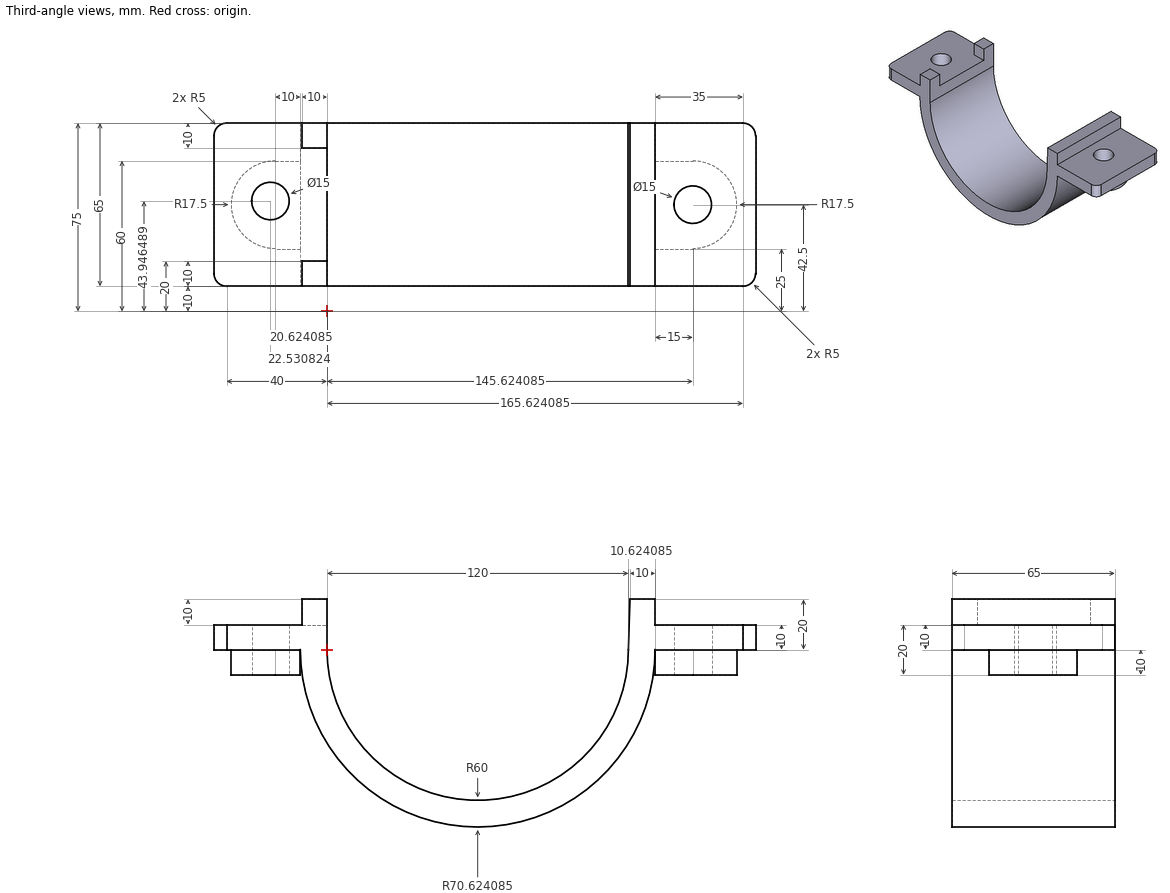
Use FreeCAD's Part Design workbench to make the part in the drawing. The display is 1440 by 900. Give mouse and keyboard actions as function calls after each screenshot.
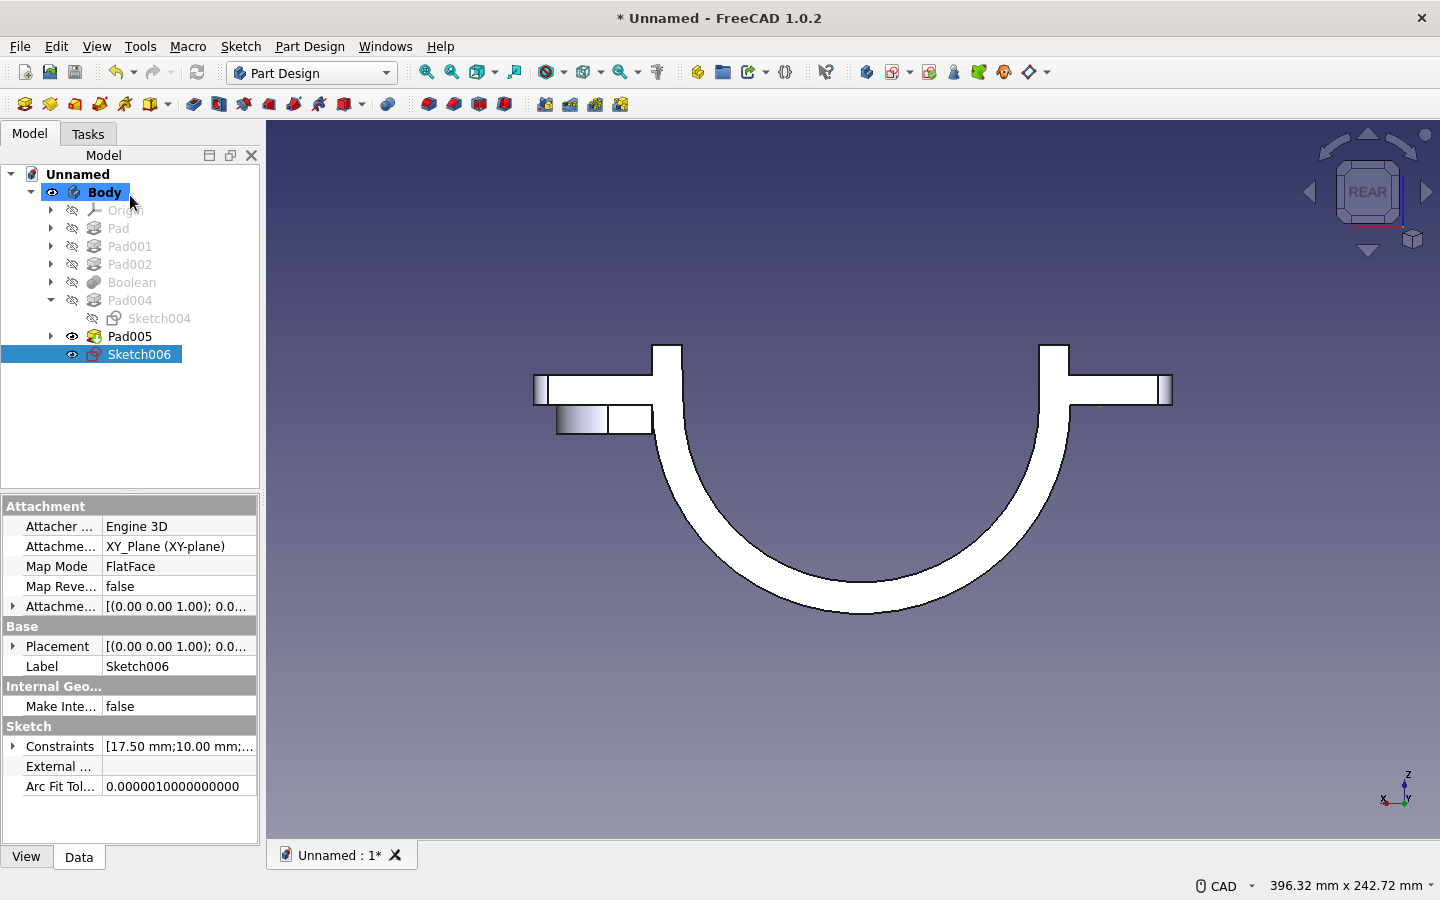
click(25, 104)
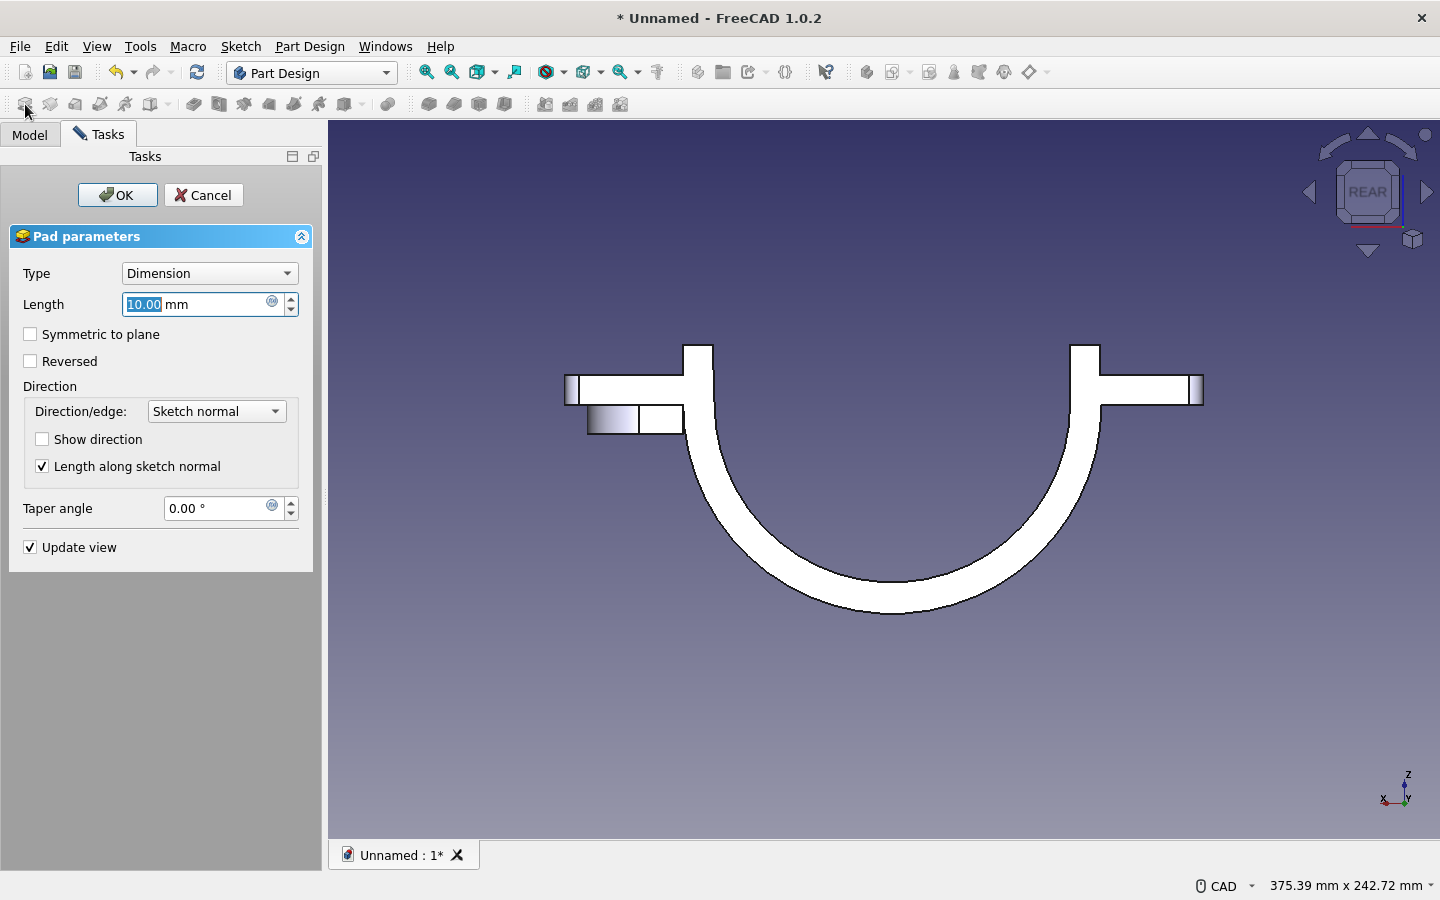
text(10)
key(Tab)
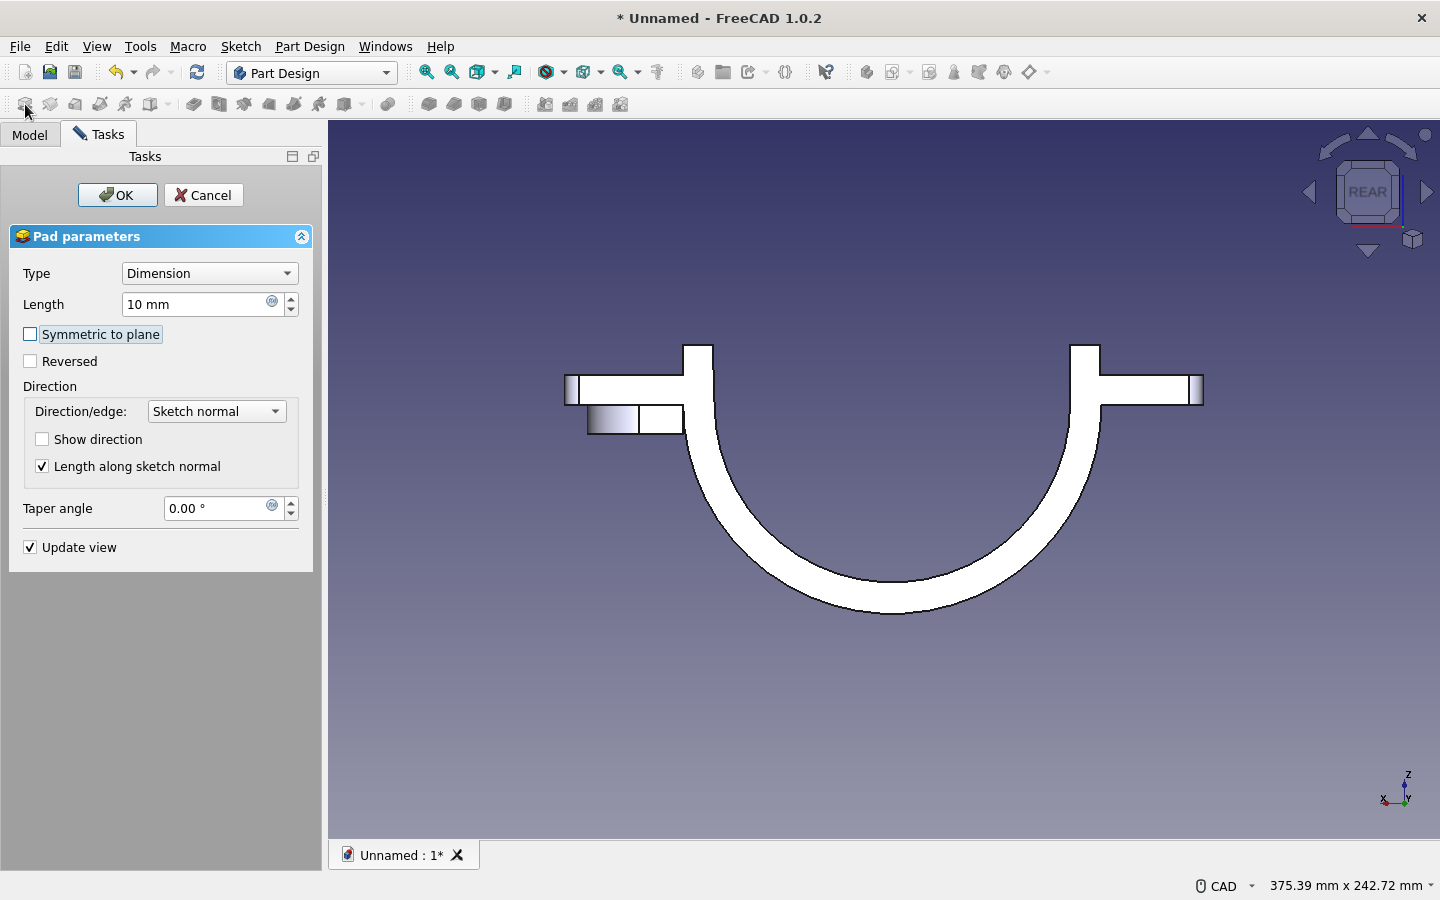
click(31, 361)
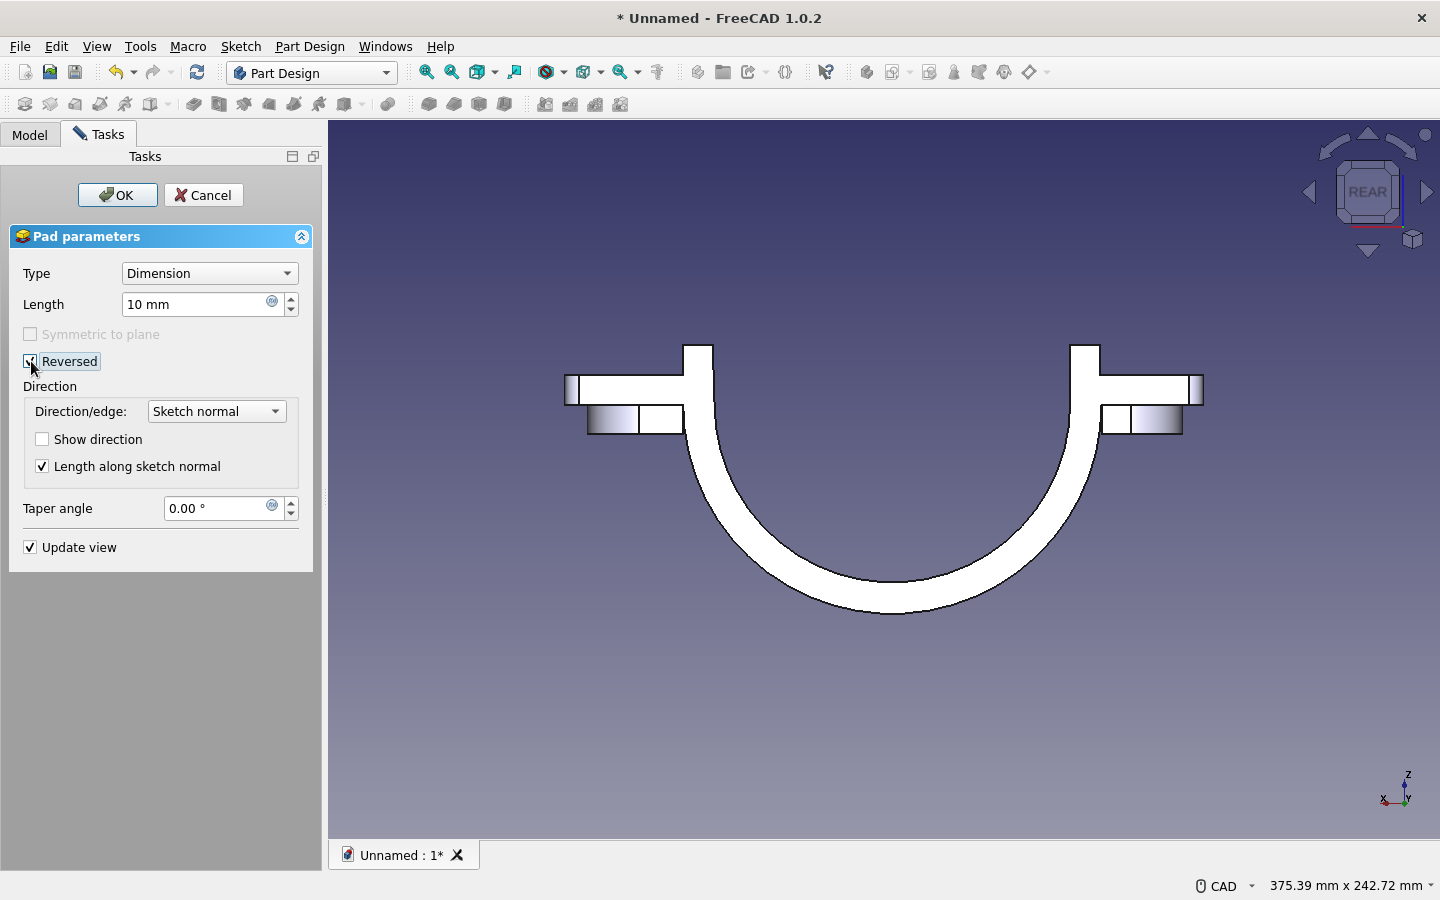
click(118, 195)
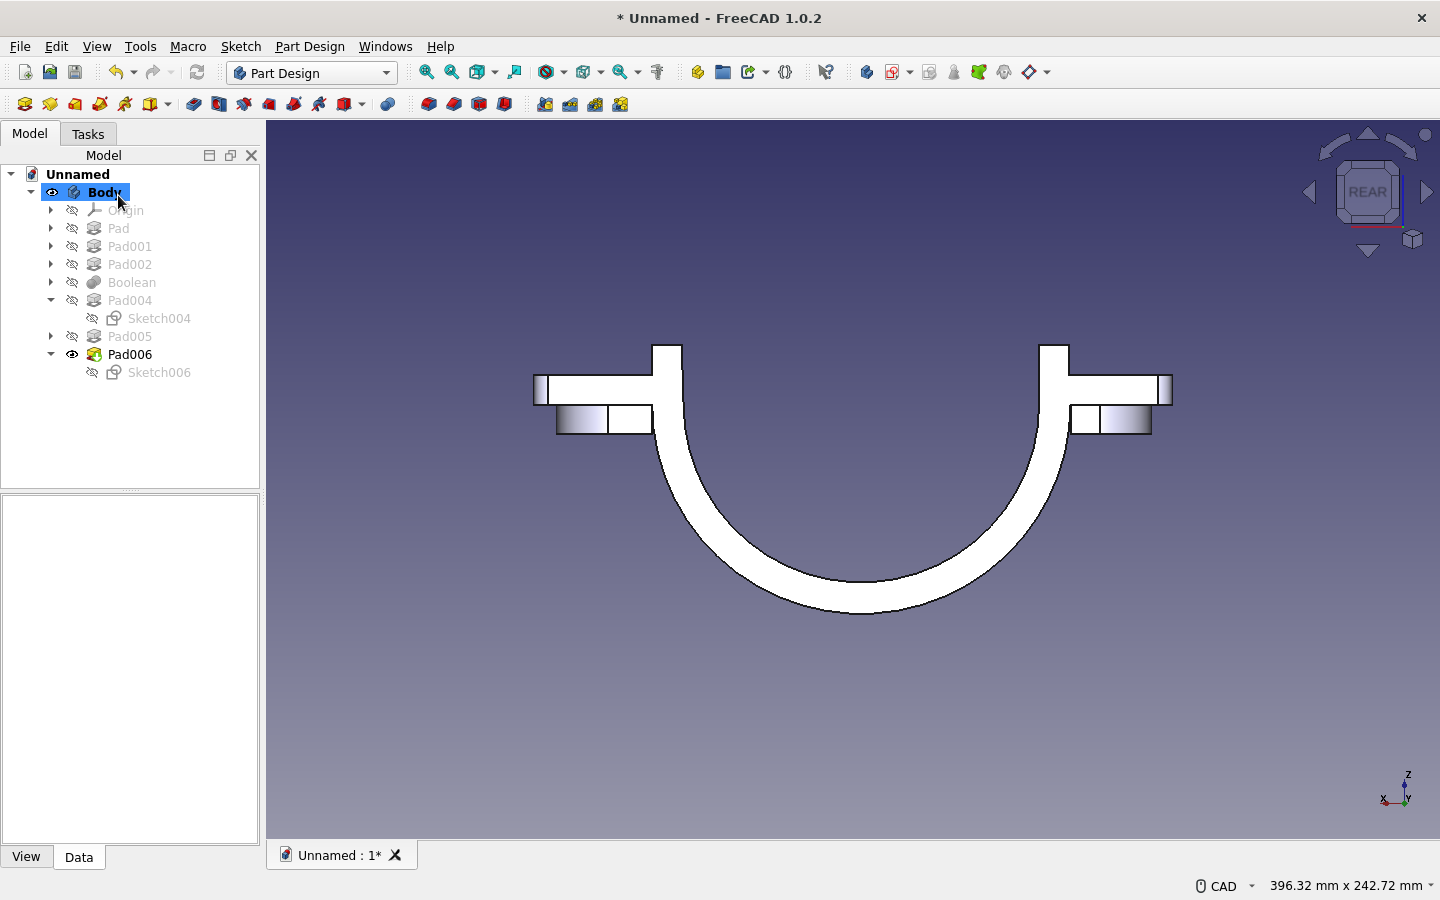
key(5)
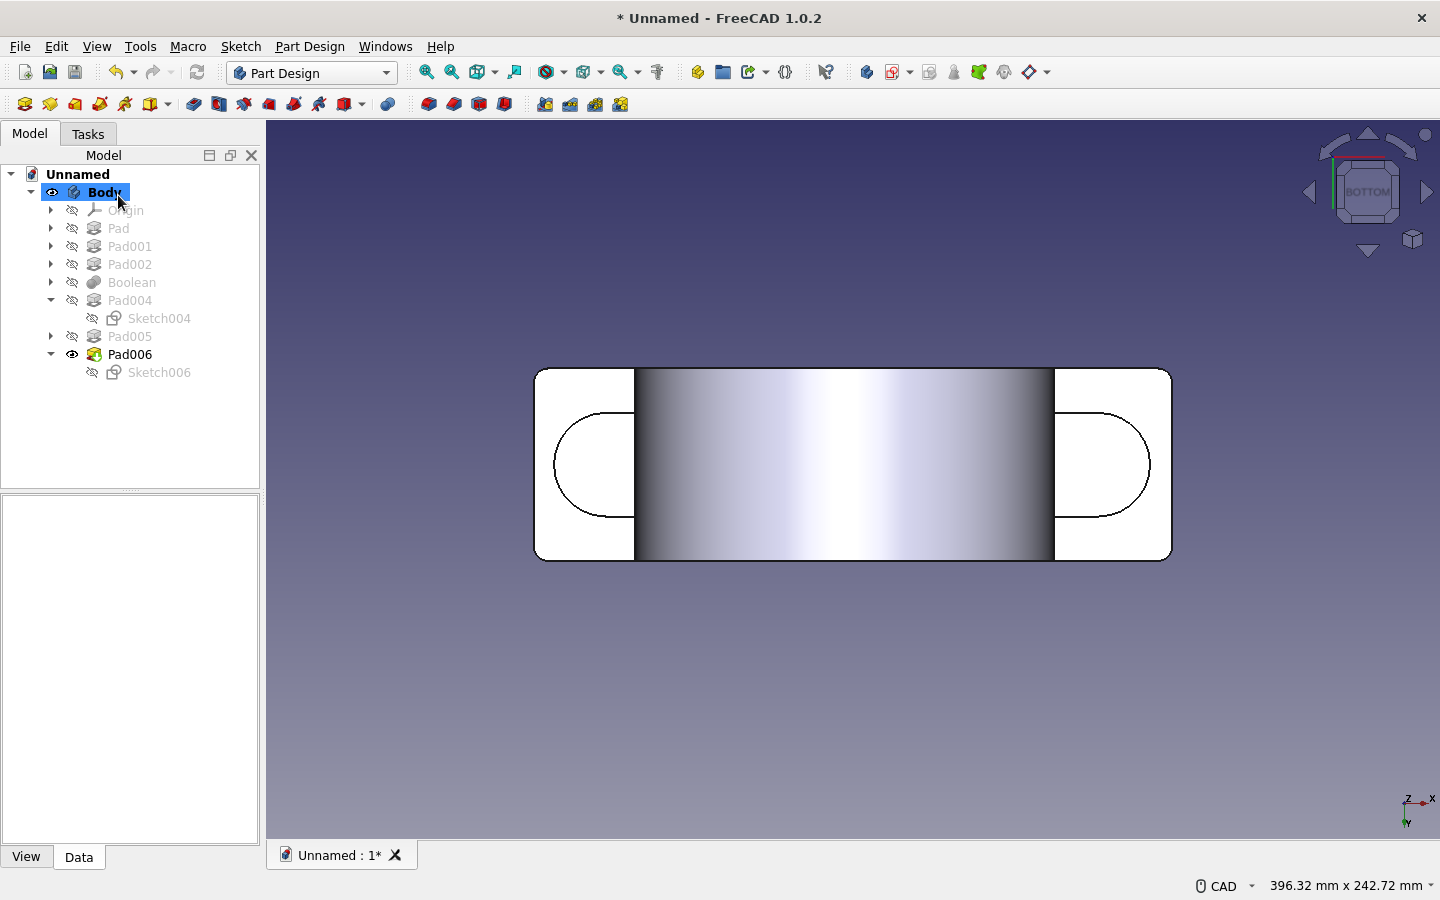
click(1102, 464)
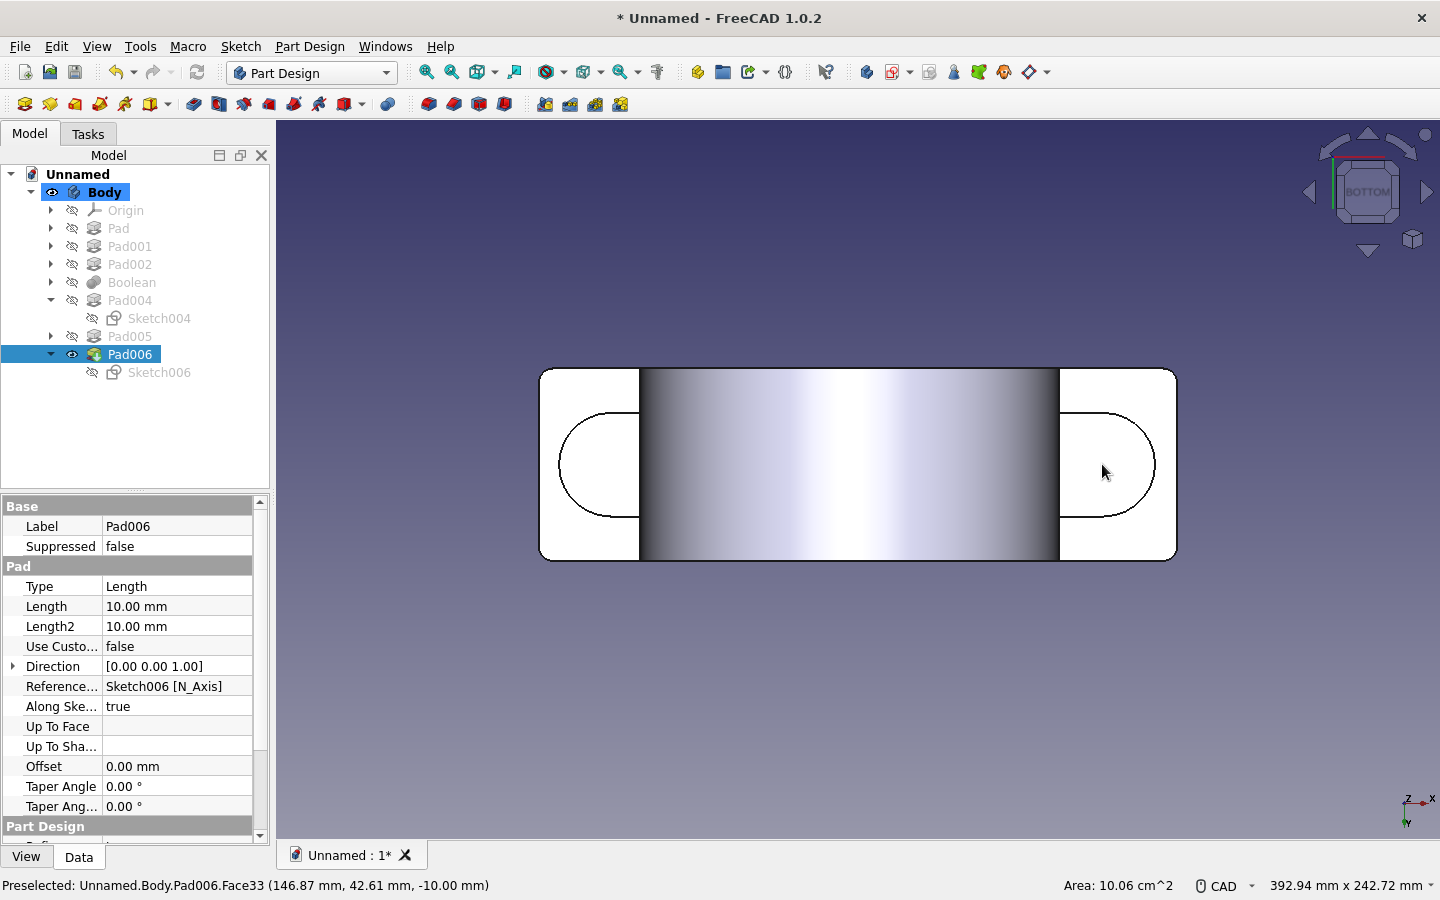
click(892, 72)